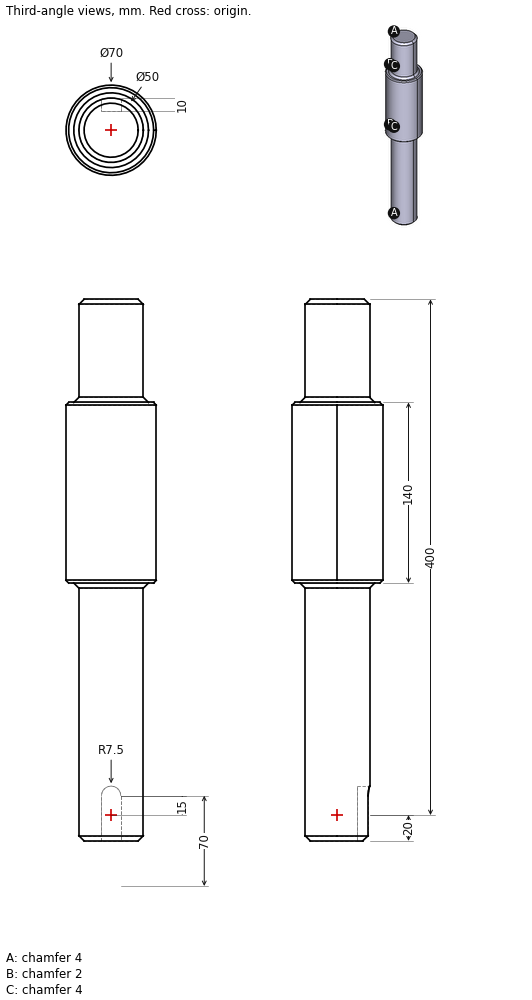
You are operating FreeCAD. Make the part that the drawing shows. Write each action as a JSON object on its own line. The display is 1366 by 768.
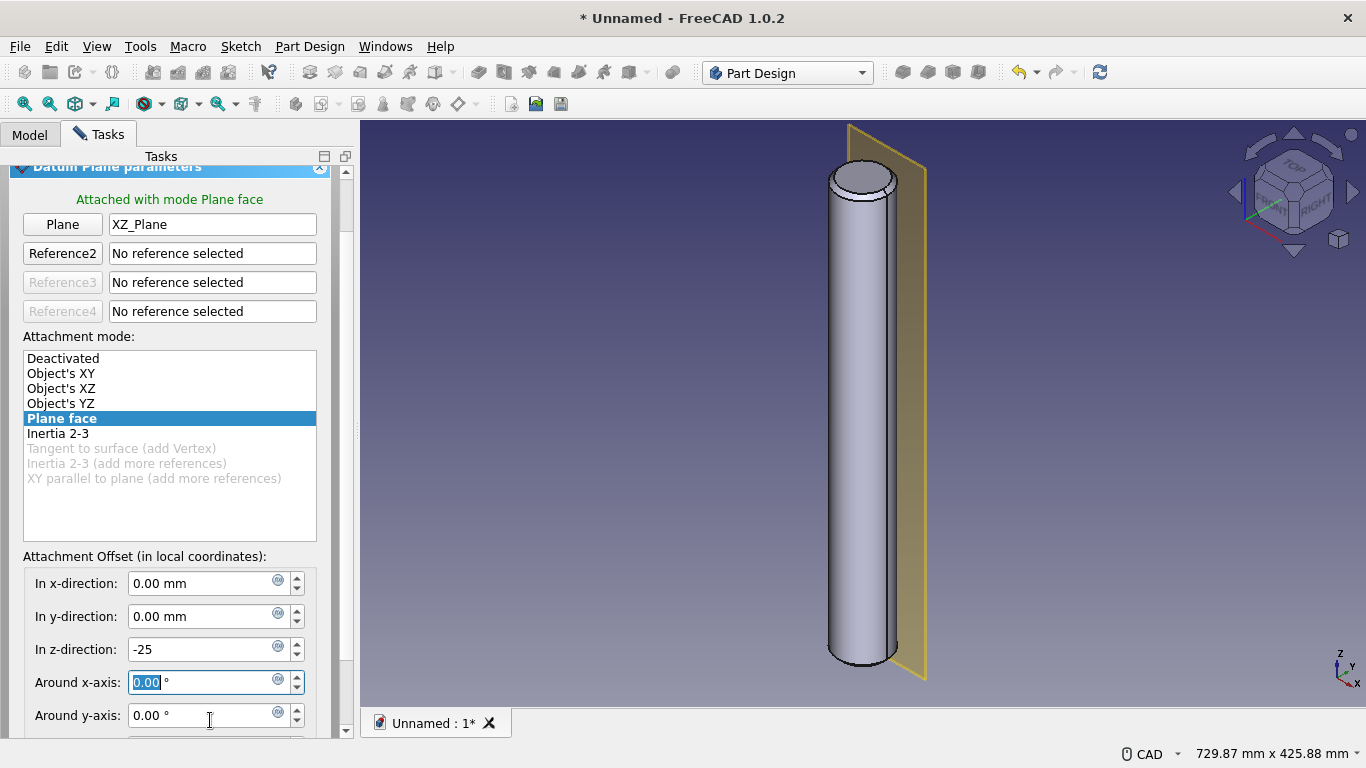
{"action": "scroll", "coordinate": [346, 452], "scroll_direction": "up", "scroll_amount": 2}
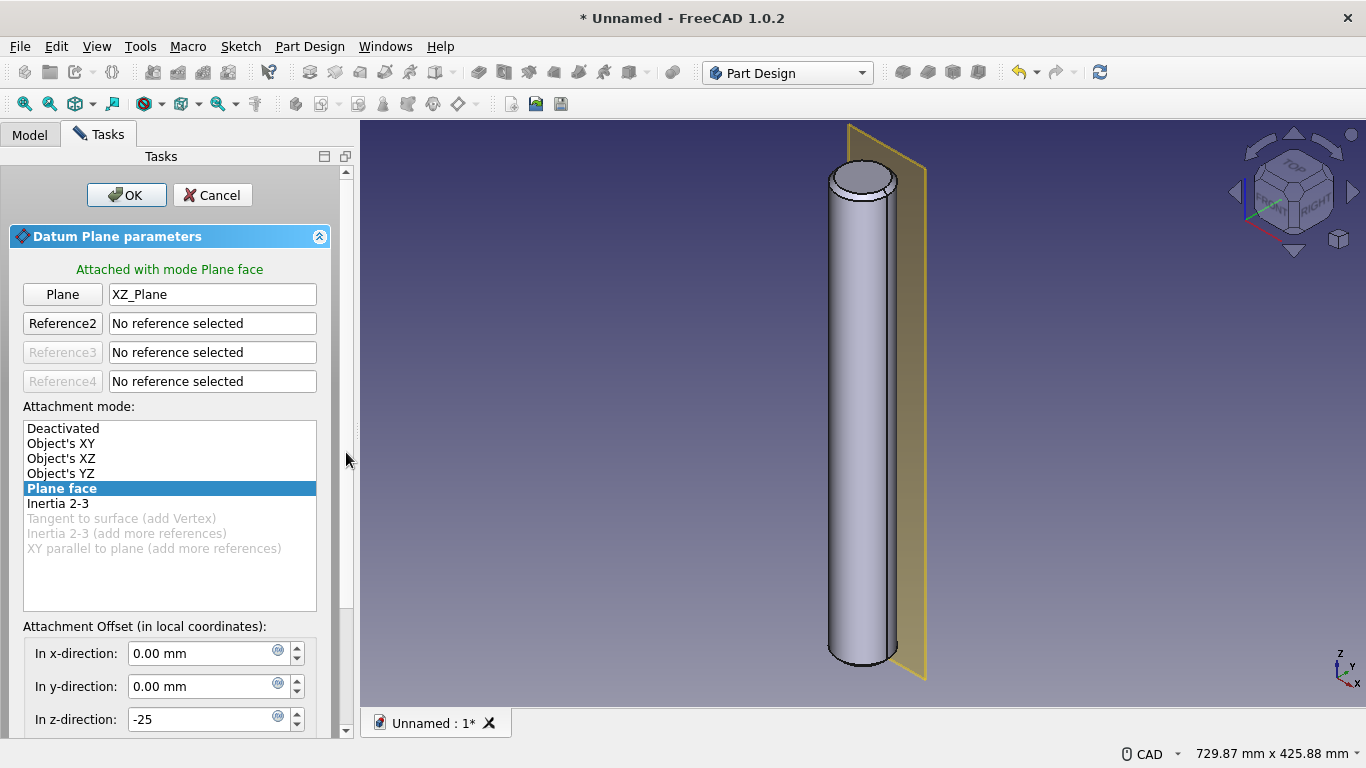
{"action": "left_click", "coordinate": [127, 195]}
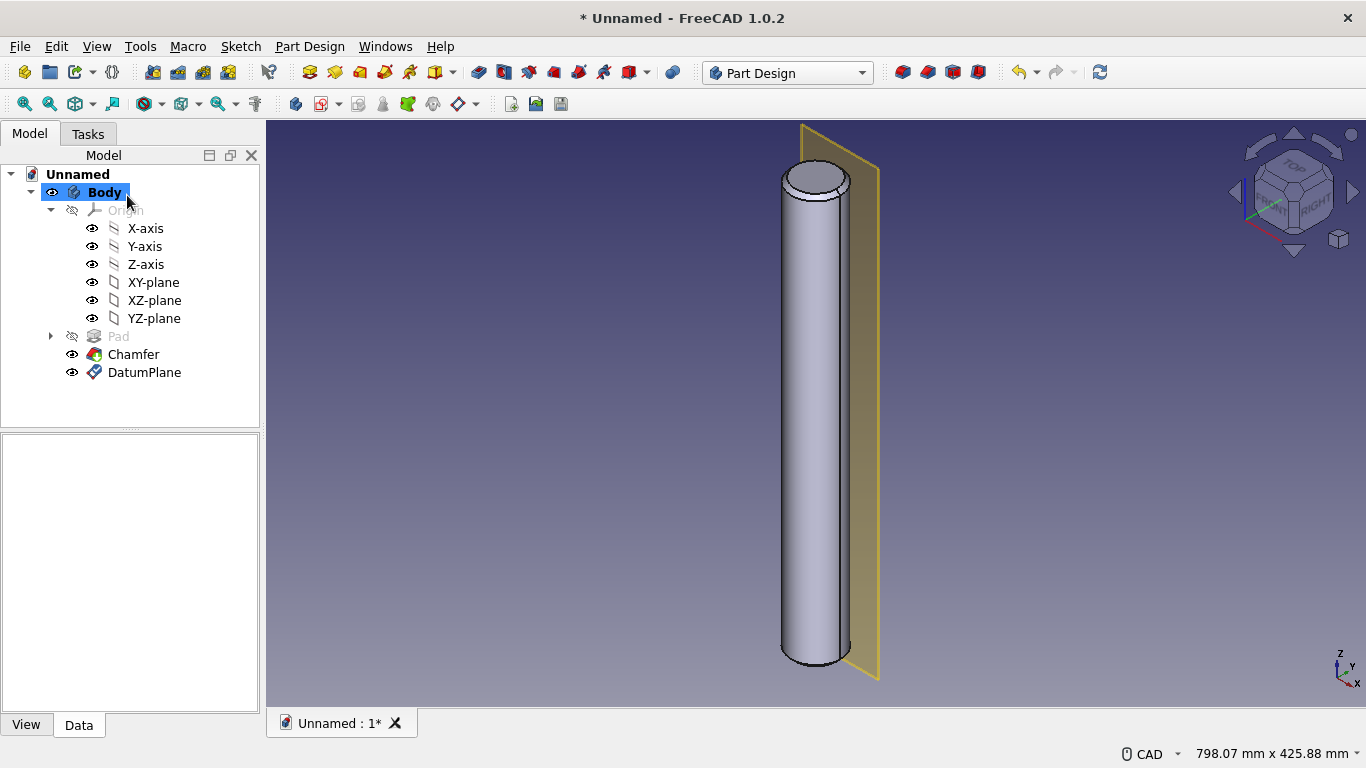
{"action": "left_click", "coordinate": [117, 372]}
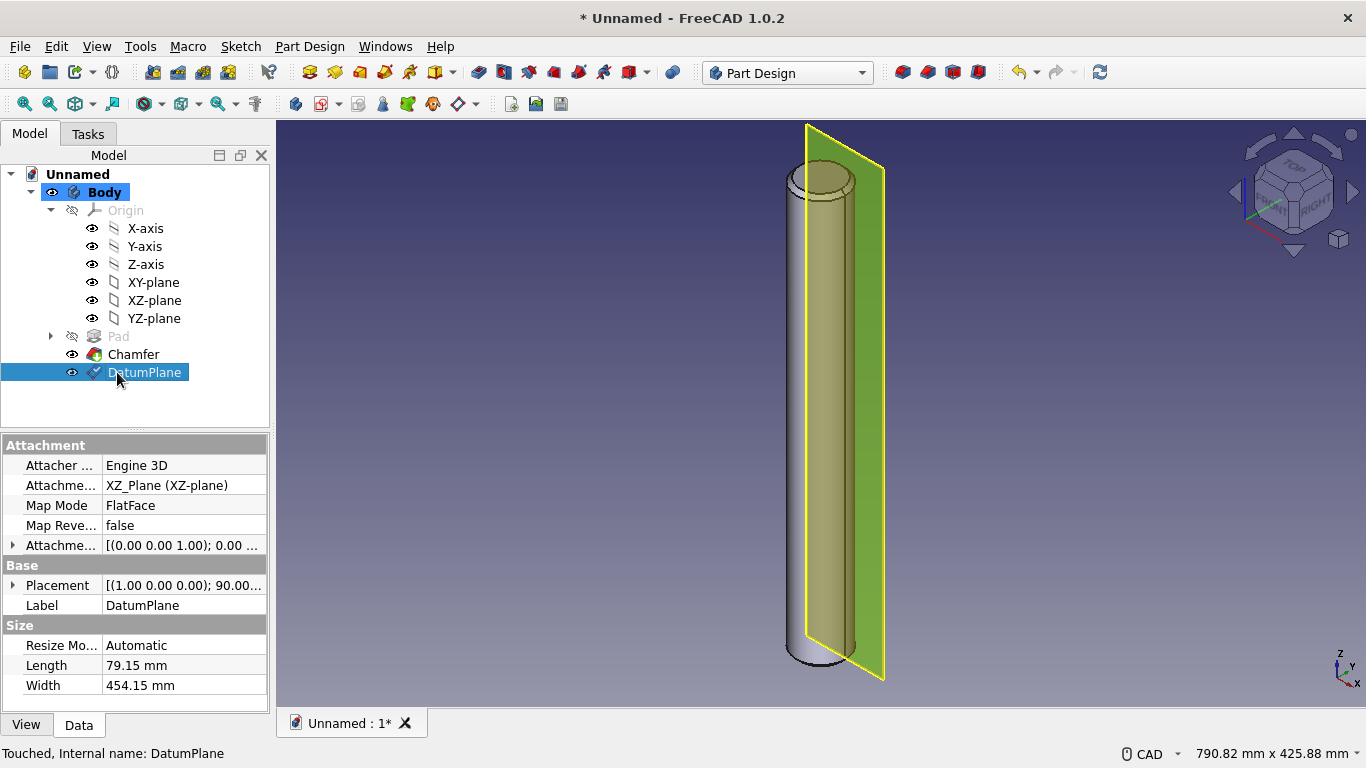
{"action": "left_click", "coordinate": [320, 104]}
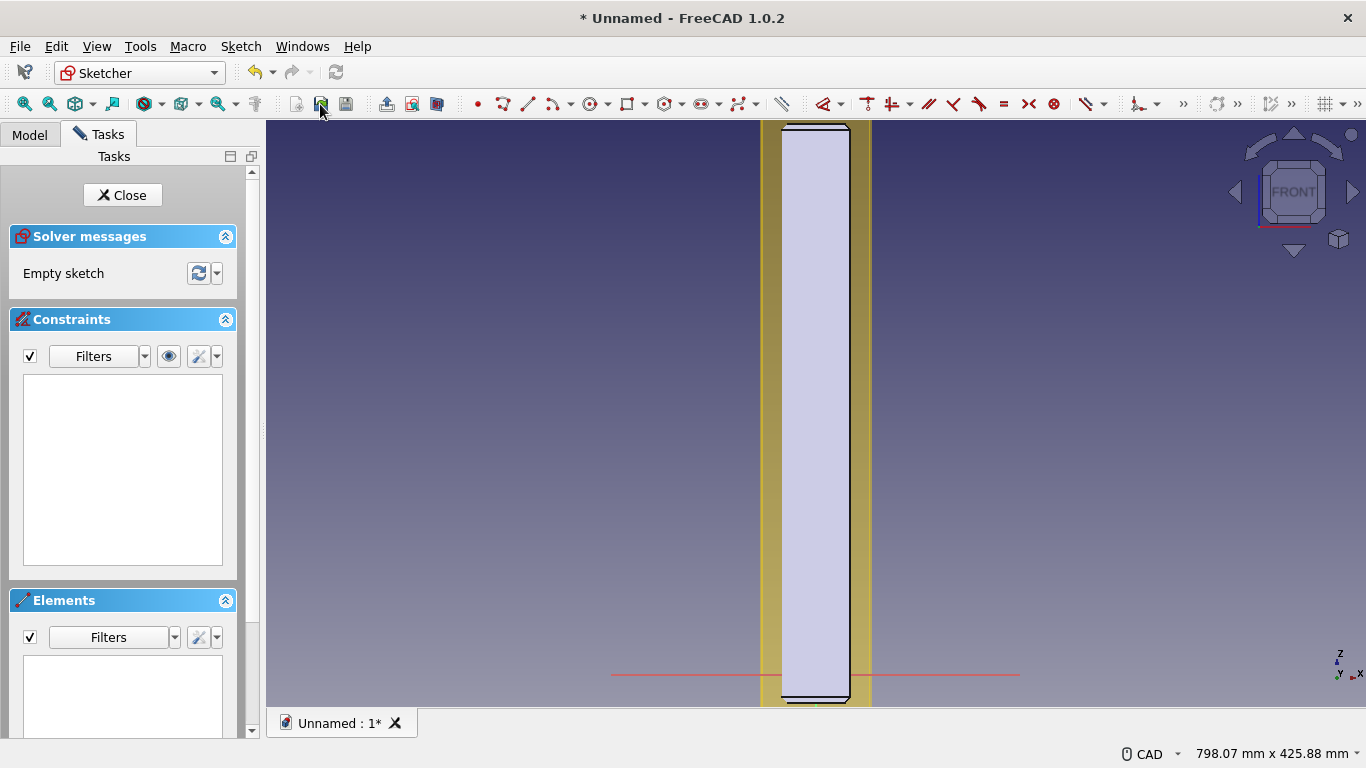
{"action": "left_click", "coordinate": [437, 104]}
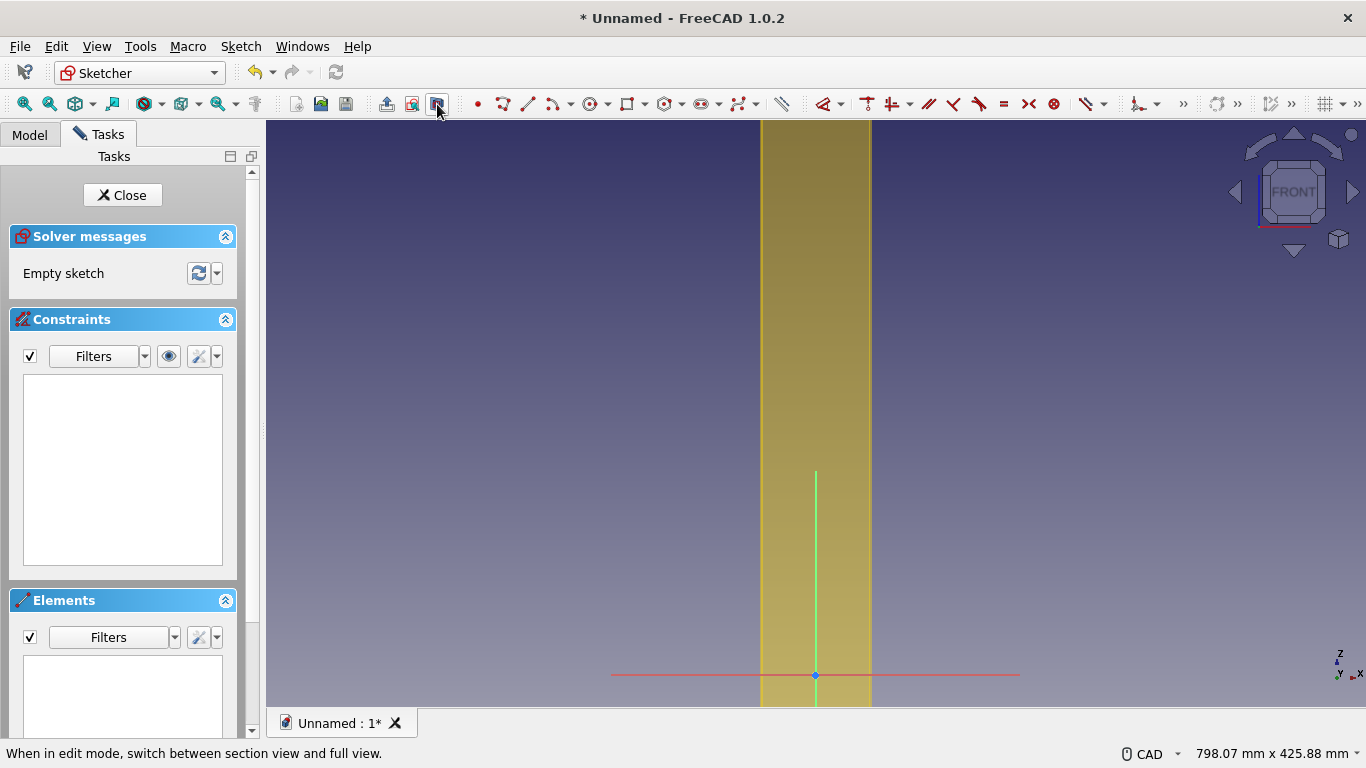
{"action": "scroll", "coordinate": [748, 414], "scroll_direction": "down", "scroll_amount": 5}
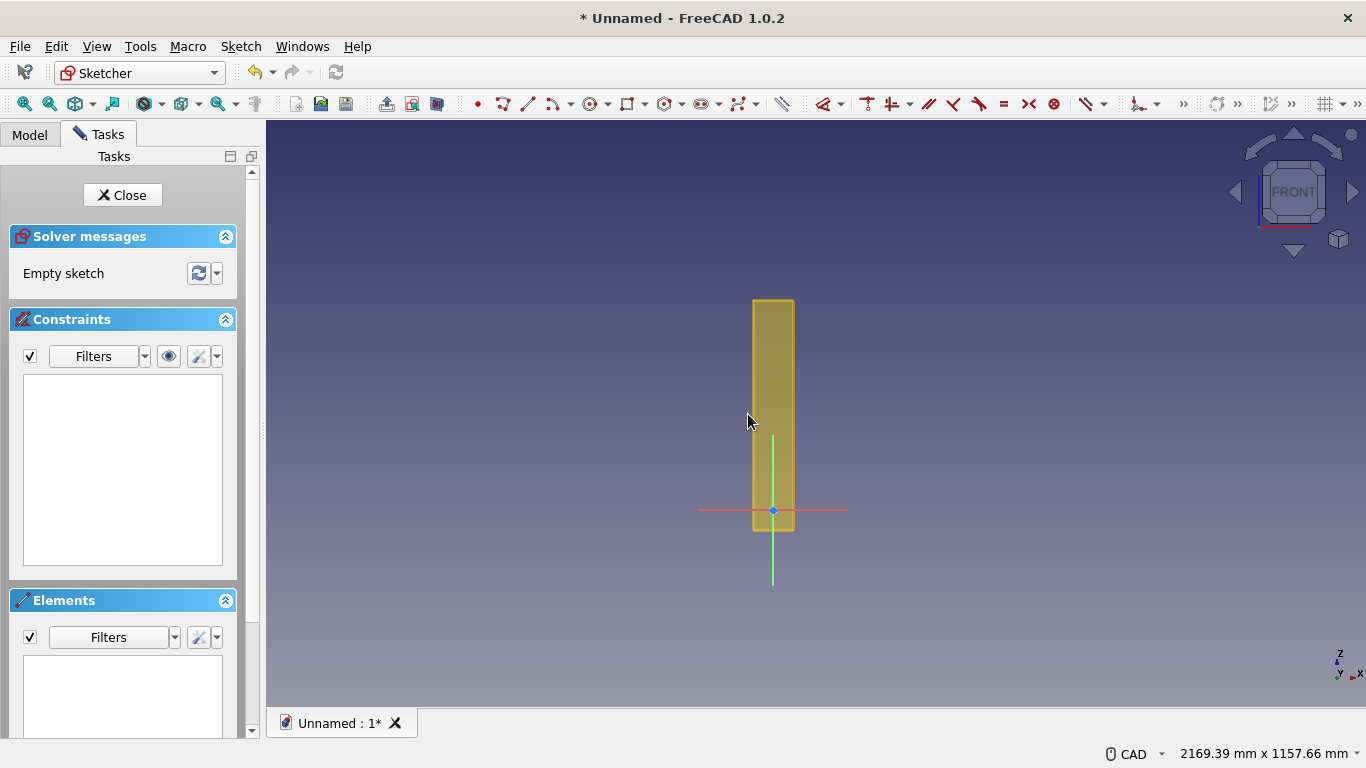
{"action": "scroll", "coordinate": [776, 532], "scroll_direction": "up", "scroll_amount": 11}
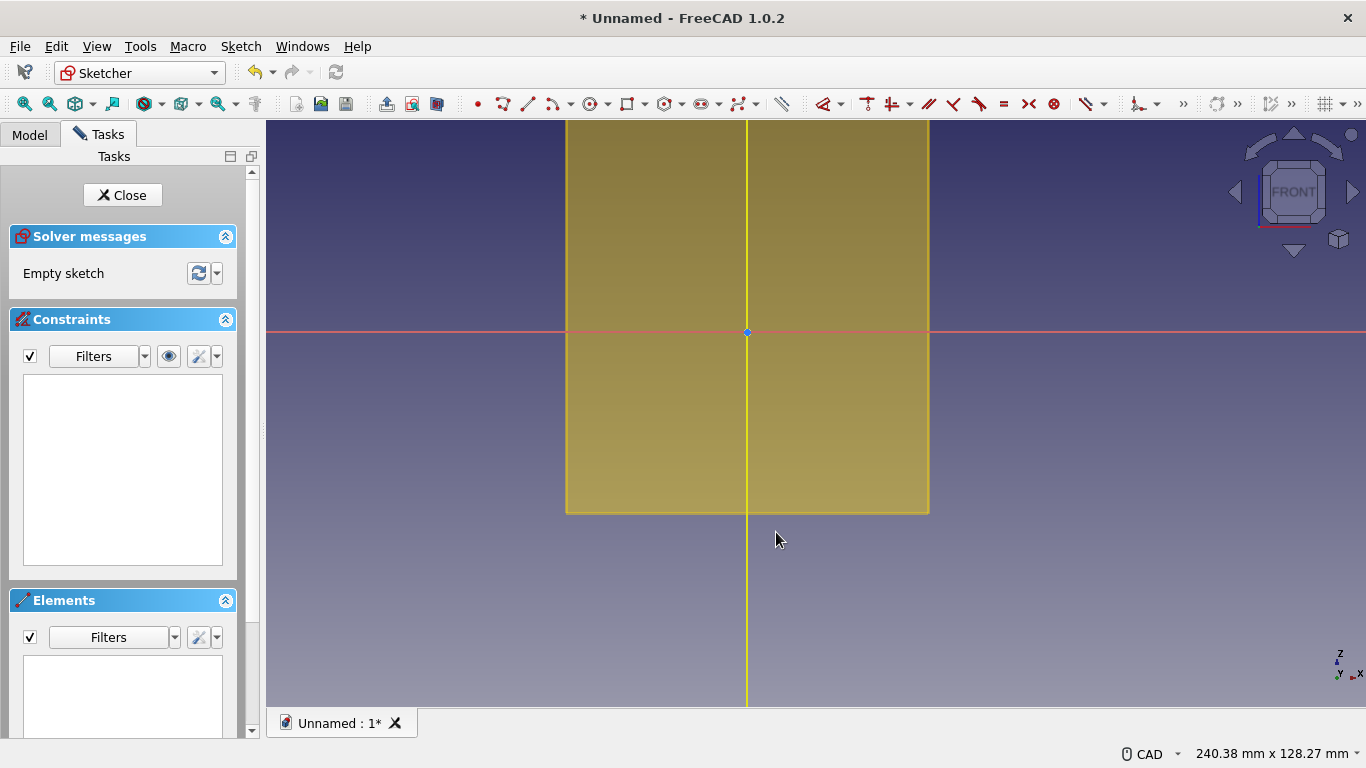
{"action": "left_click", "coordinate": [503, 104]}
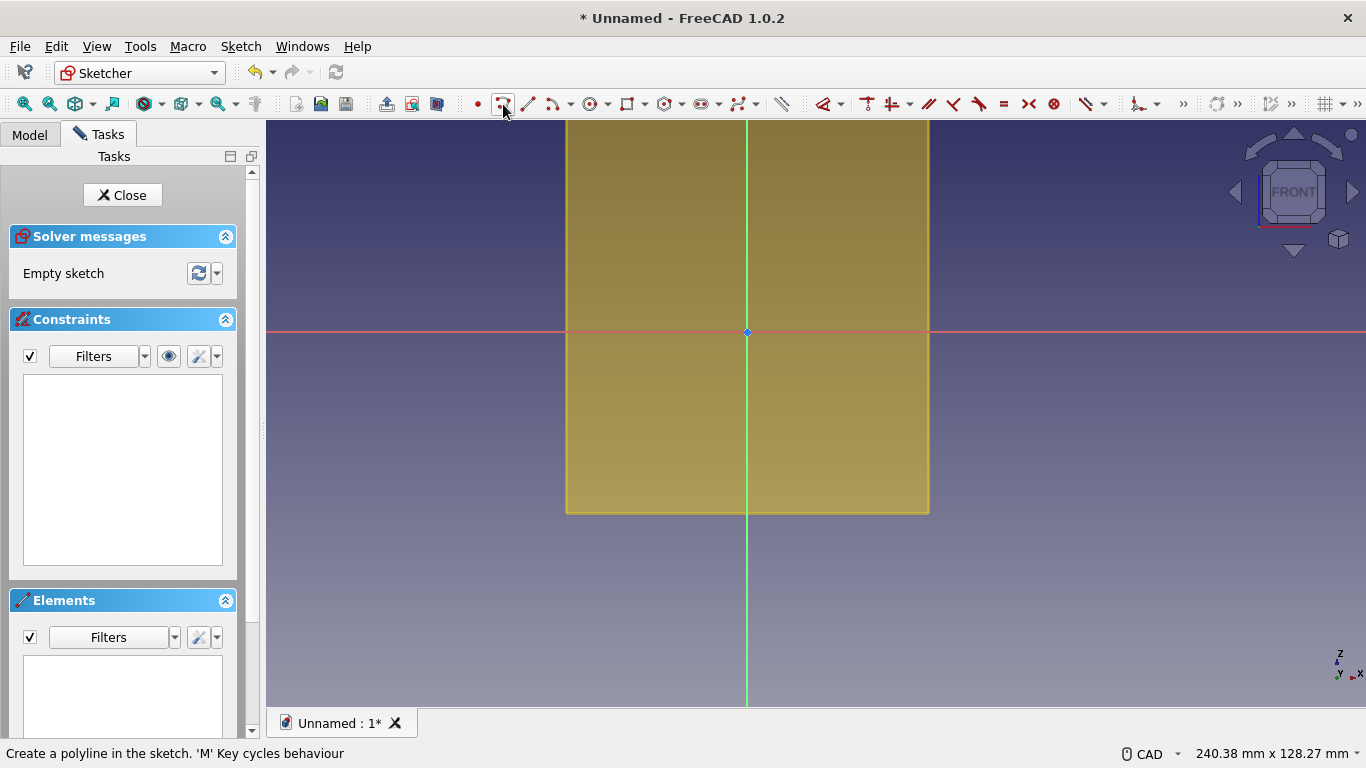
{"action": "left_click", "coordinate": [782, 263]}
{"action": "left_click", "coordinate": [782, 584]}
{"action": "left_click", "coordinate": [713, 584]}
{"action": "left_click", "coordinate": [713, 263]}
{"action": "right_click", "coordinate": [713, 263]}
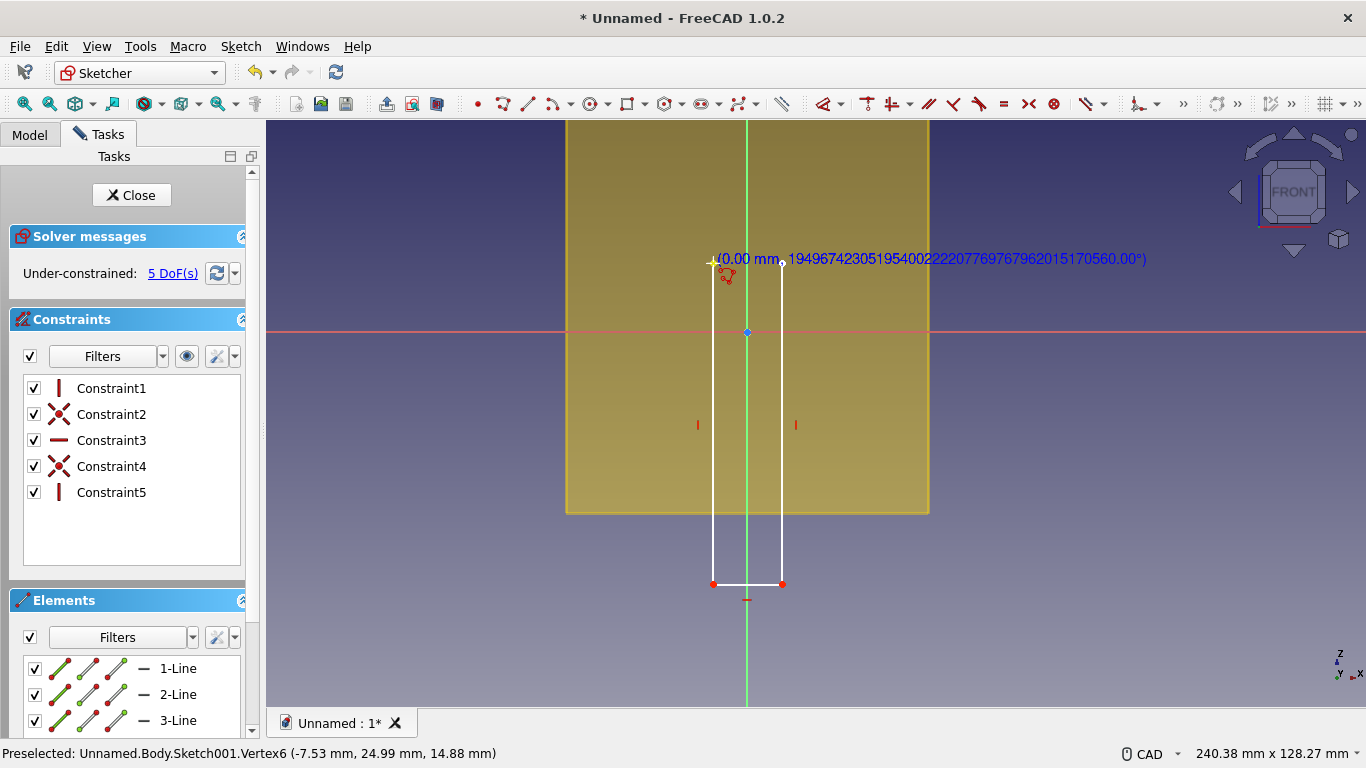
{"action": "key", "text": "g 3 a"}